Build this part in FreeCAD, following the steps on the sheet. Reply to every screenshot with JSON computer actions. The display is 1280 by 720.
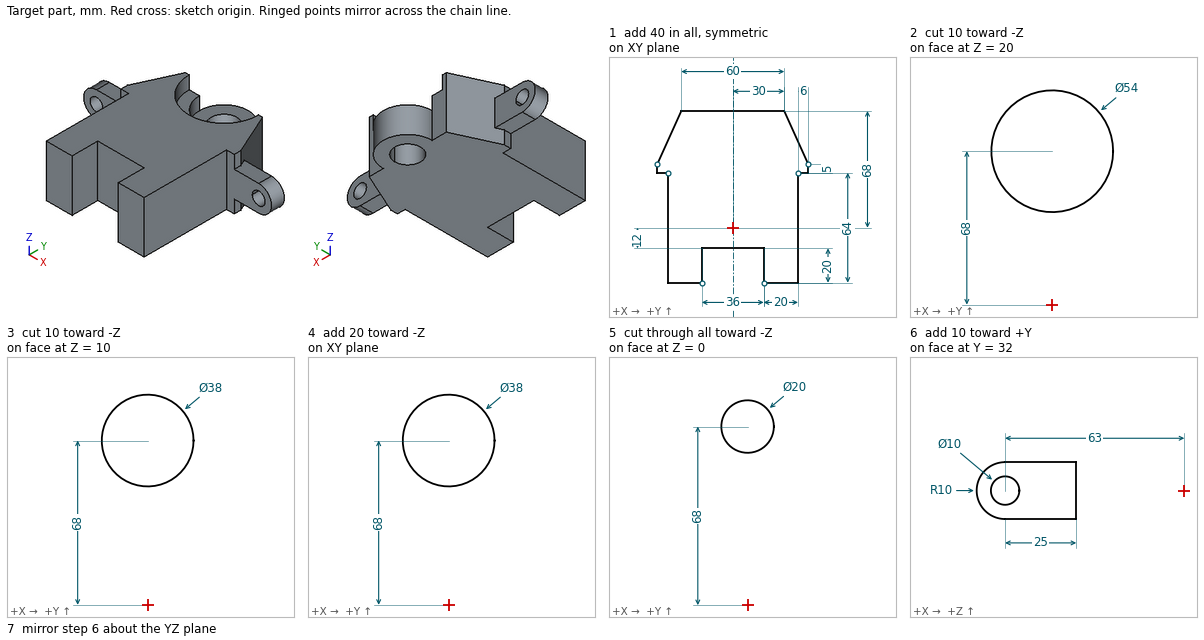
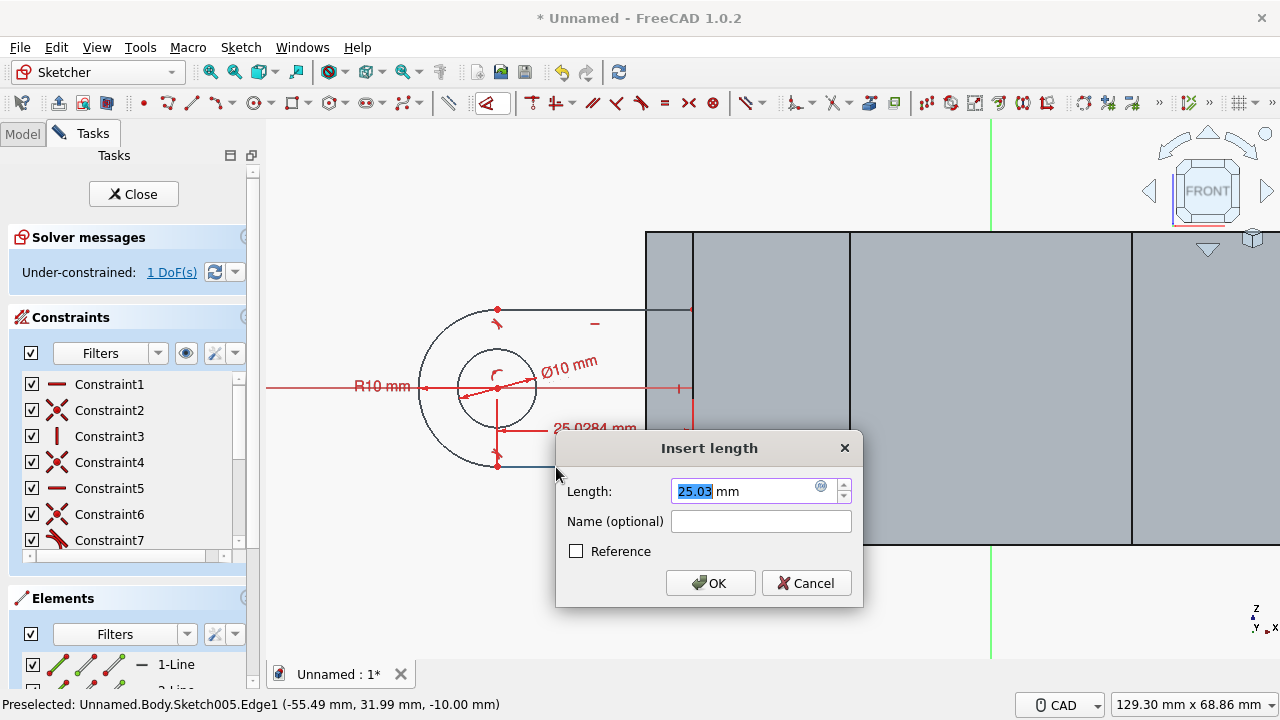
{"action": "type", "text": "25"}
{"action": "key", "text": "Return"}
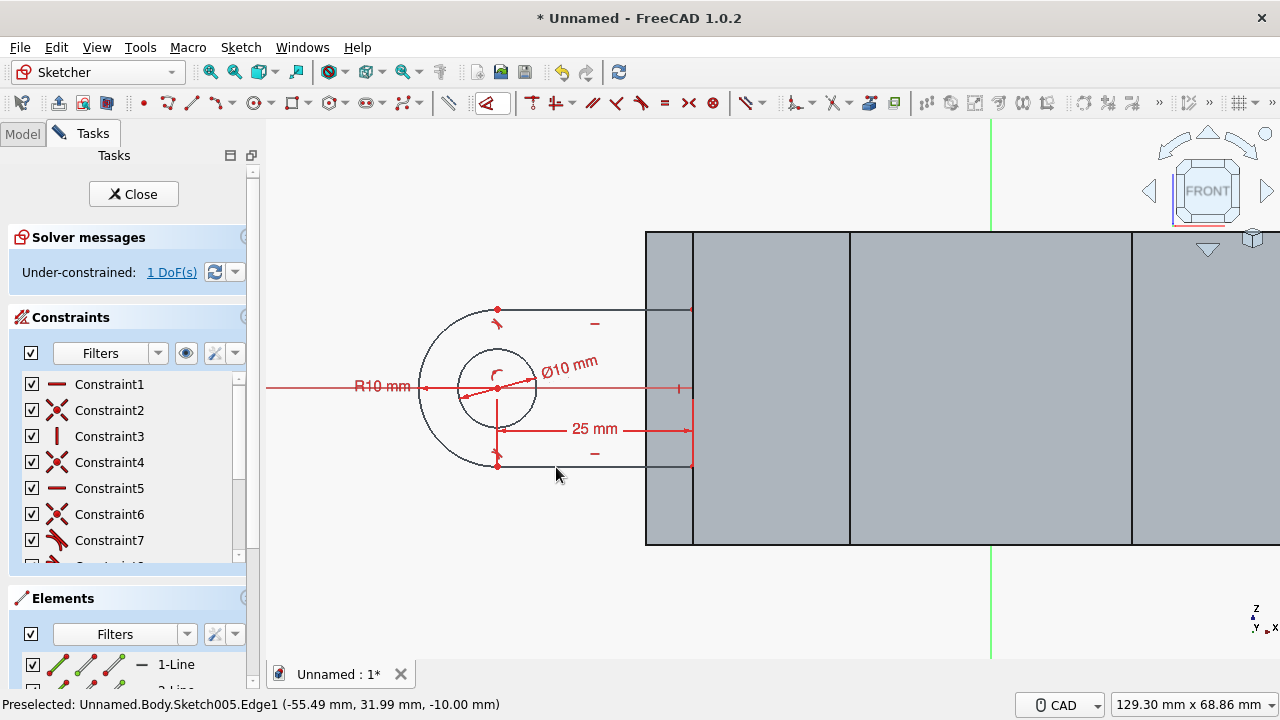
{"action": "left_click", "coordinate": [497, 388]}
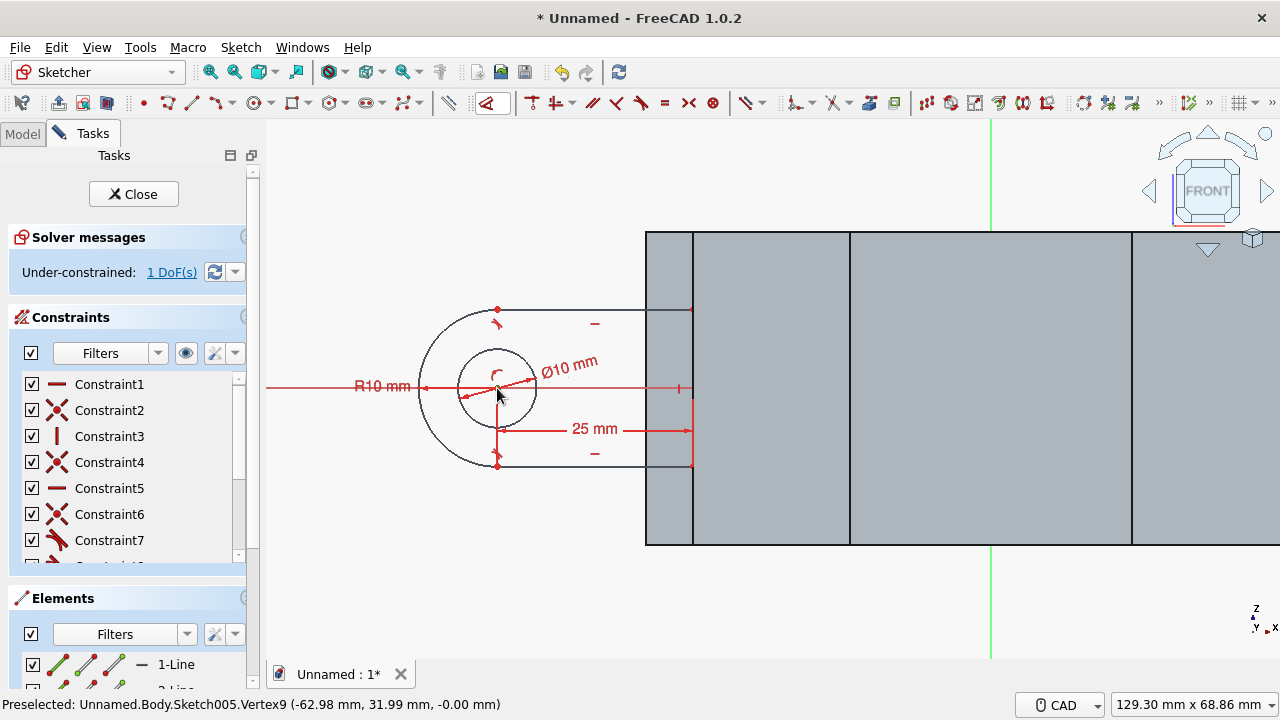
{"action": "left_click", "coordinate": [504, 104]}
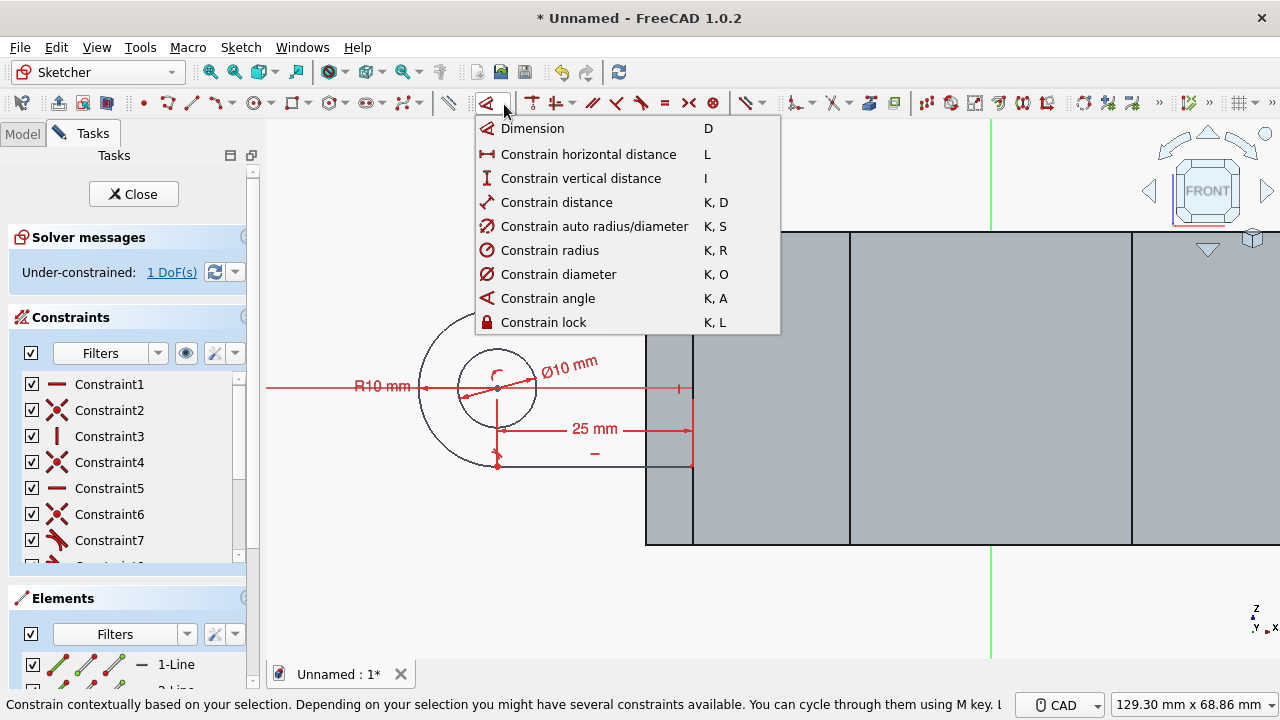
{"action": "left_click", "coordinate": [628, 154]}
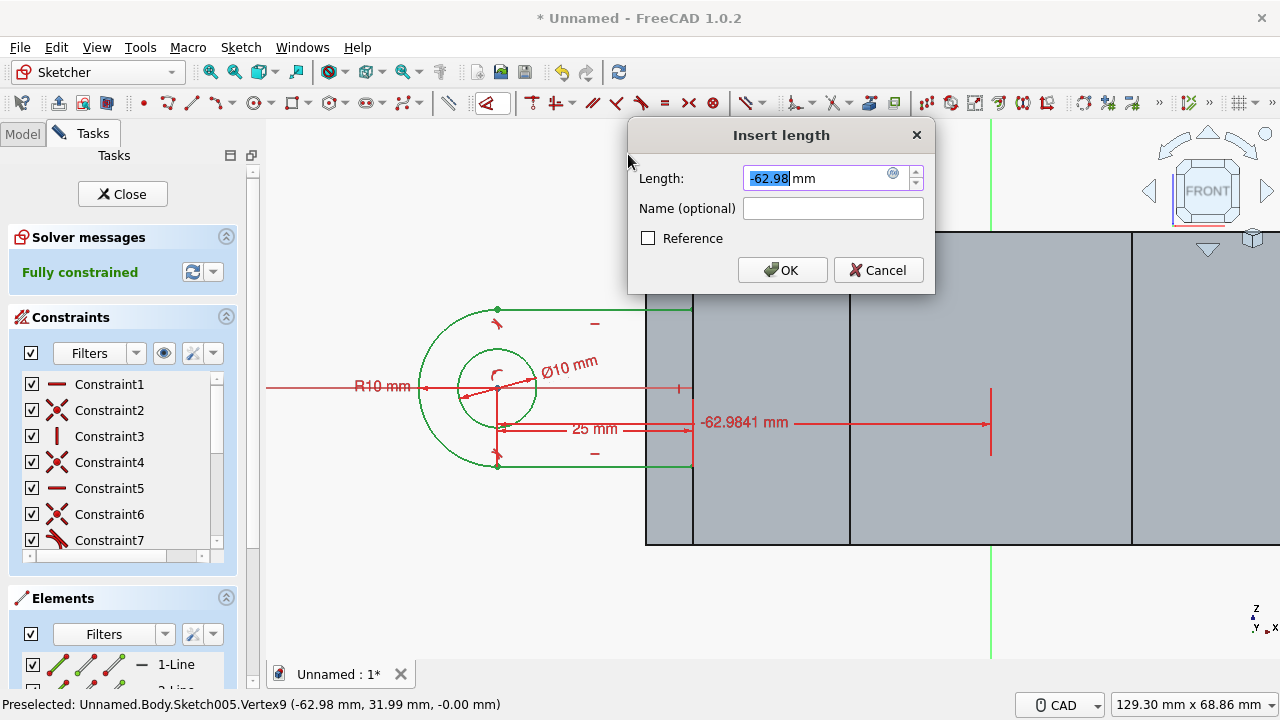
{"action": "type", "text": "-63"}
{"action": "key", "text": "Return"}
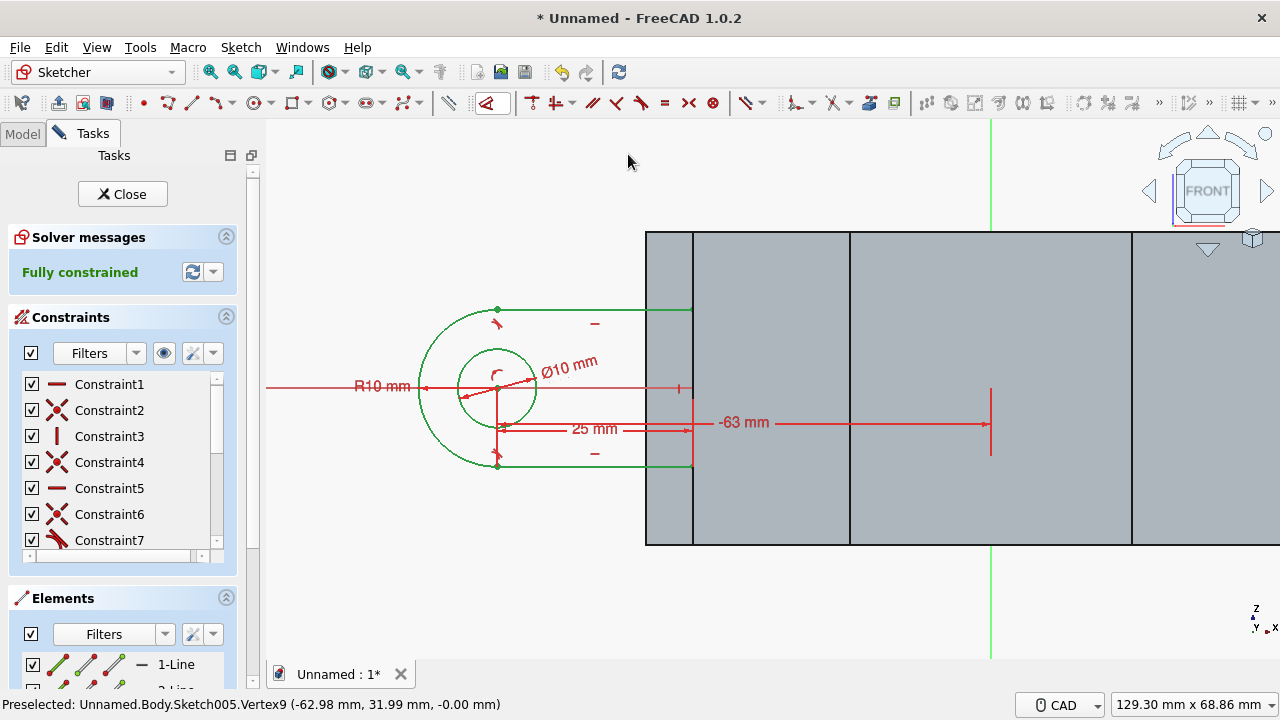
{"action": "left_click", "coordinate": [123, 194]}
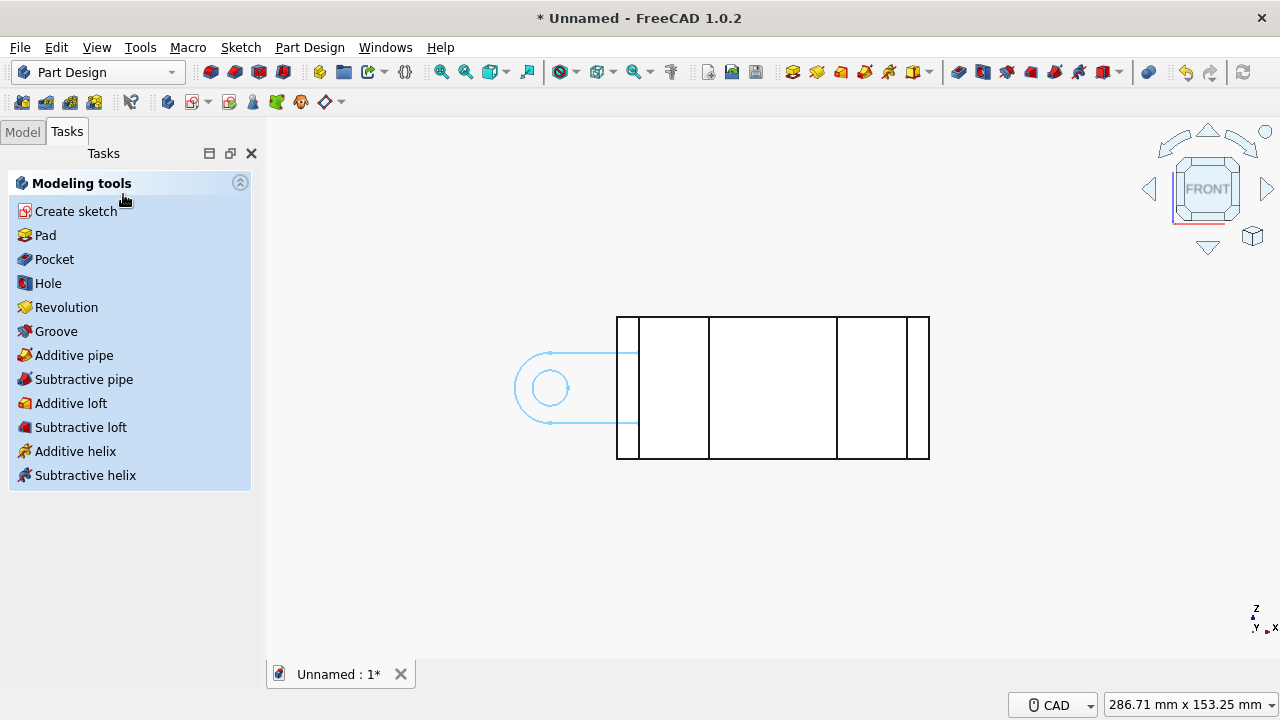
{"action": "left_click", "coordinate": [794, 72]}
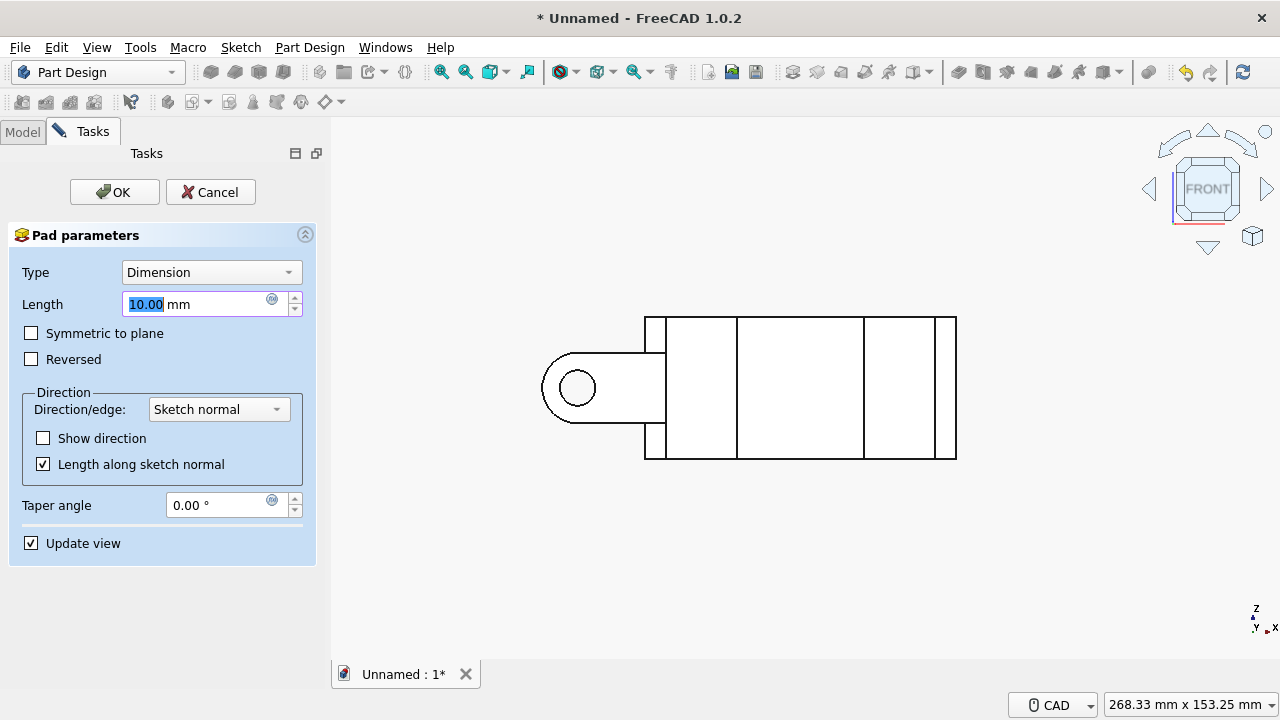
{"action": "type", "text": "10"}
{"action": "key", "text": "Tab"}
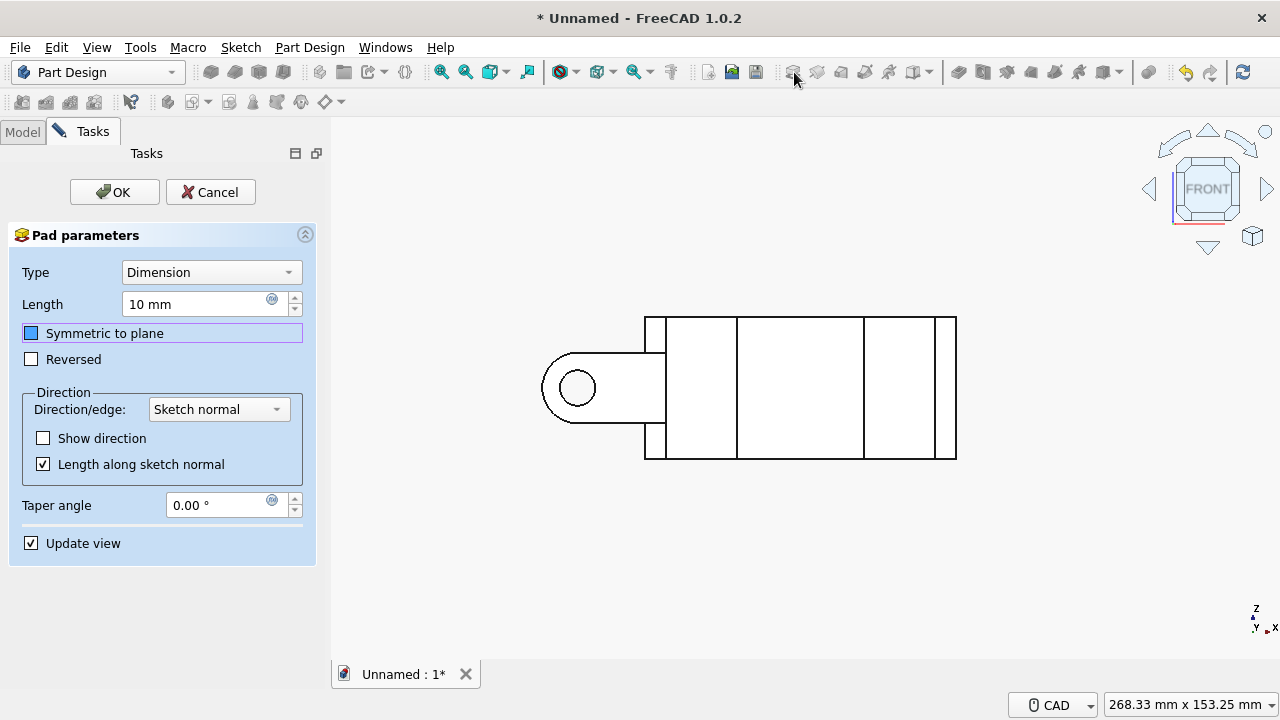
{"action": "left_click", "coordinate": [30, 359]}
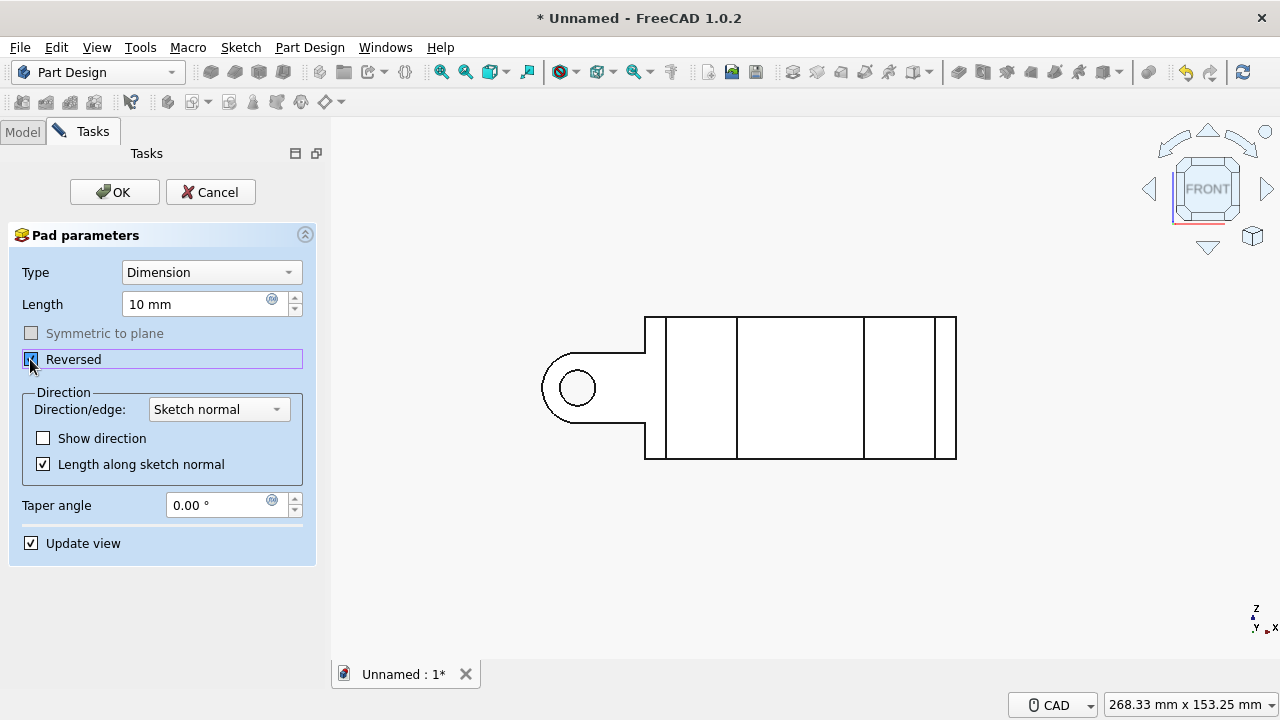
{"action": "left_click", "coordinate": [115, 192]}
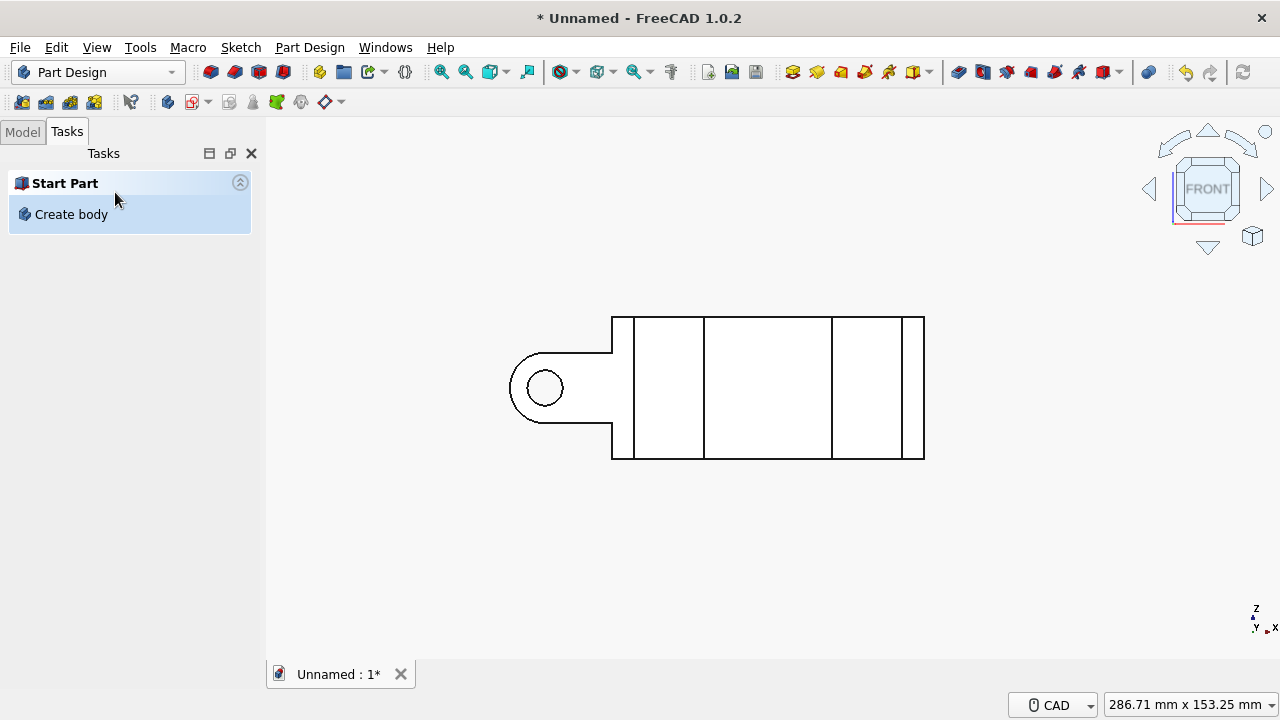
{"action": "left_click", "coordinate": [442, 72]}